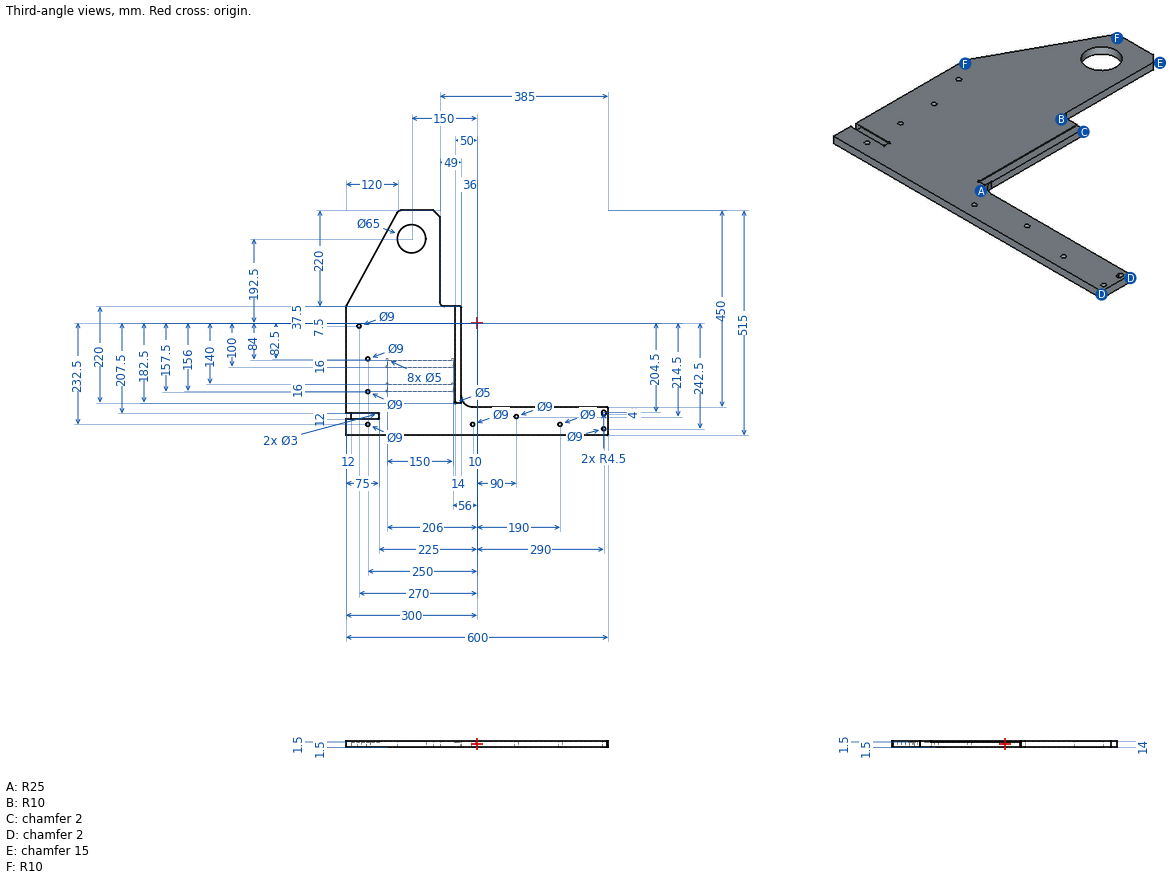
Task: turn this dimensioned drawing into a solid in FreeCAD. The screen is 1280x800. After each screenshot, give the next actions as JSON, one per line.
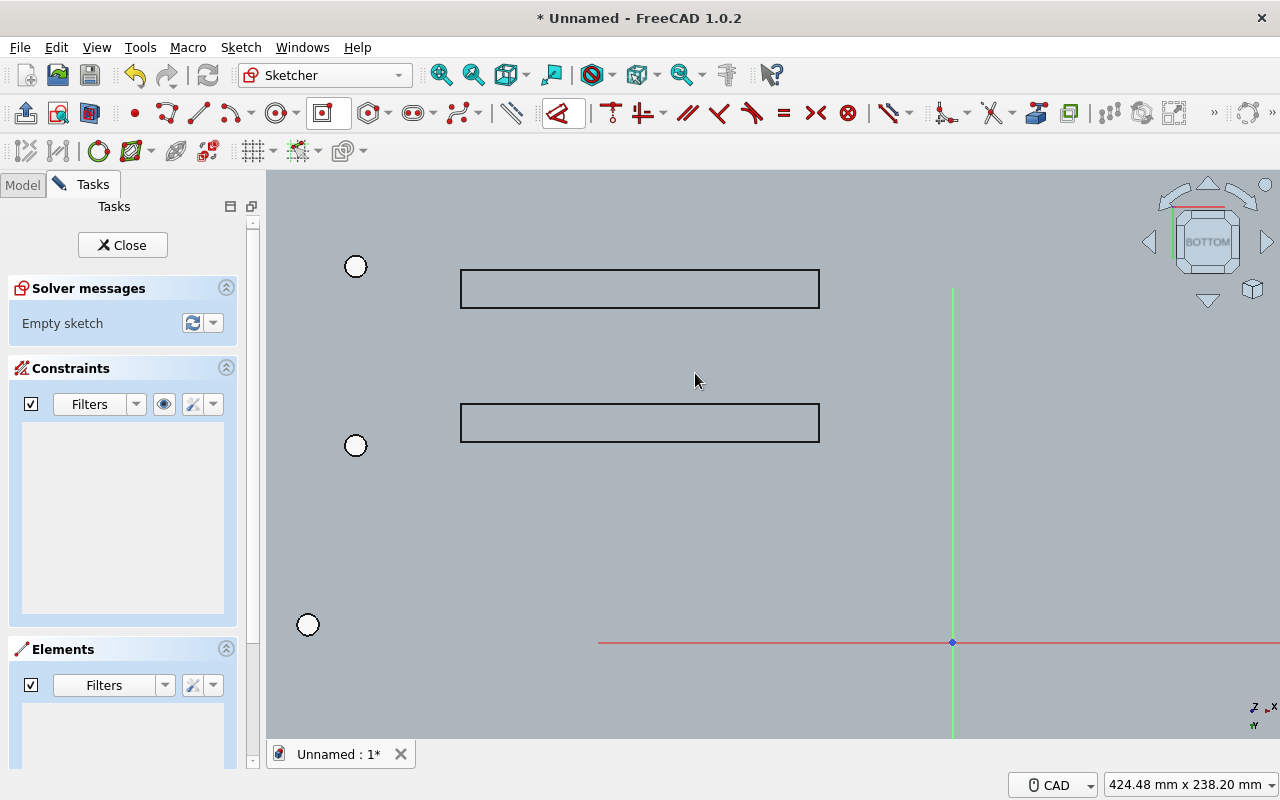
{"action": "left_click", "coordinate": [276, 114]}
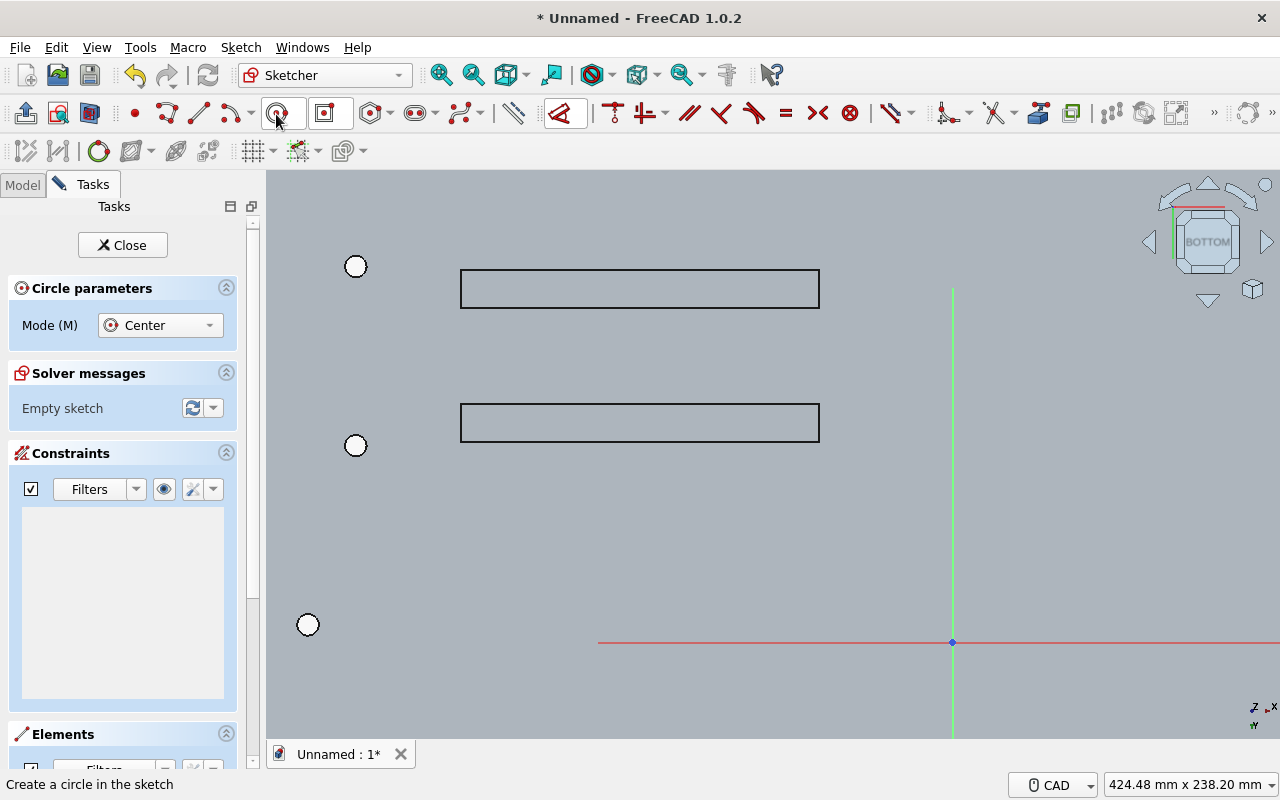
{"action": "scroll", "coordinate": [461, 442], "scroll_direction": "up", "scroll_amount": 7}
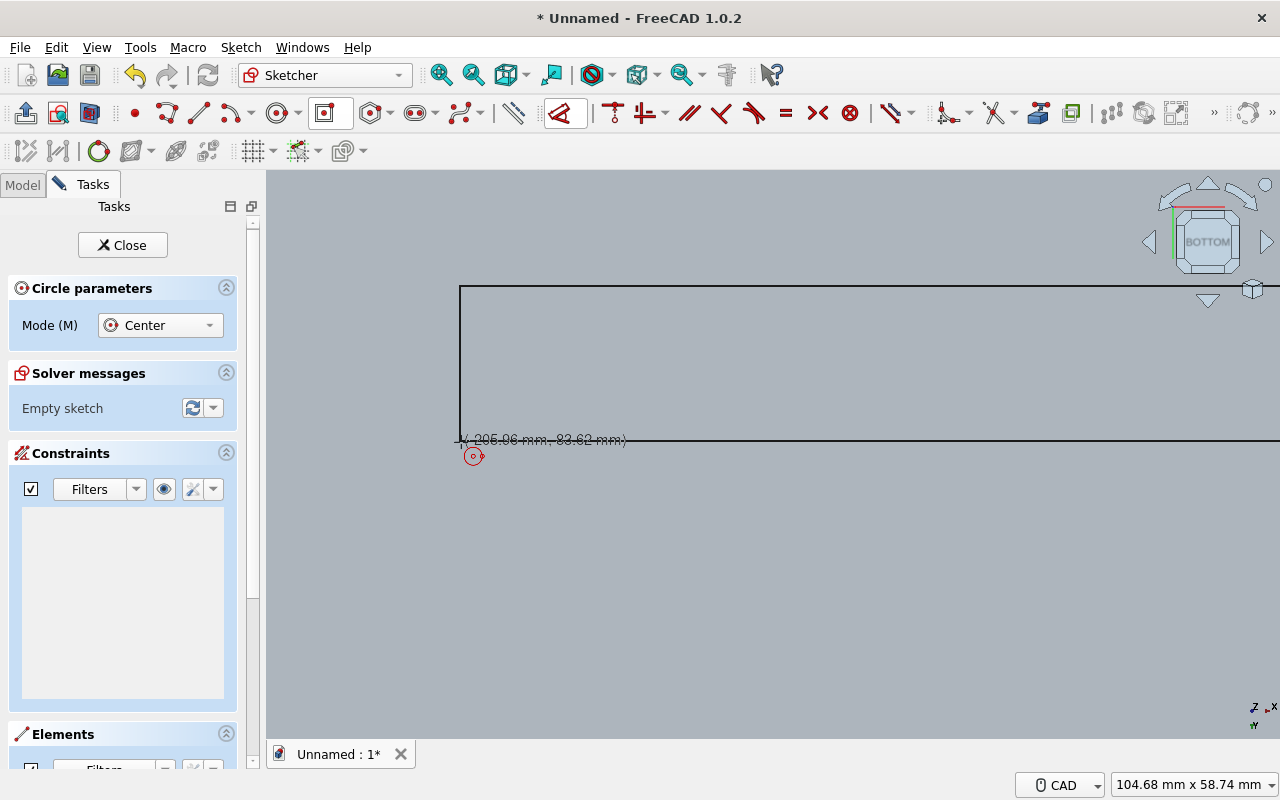
{"action": "scroll", "coordinate": [462, 444], "scroll_direction": "down", "scroll_amount": 7}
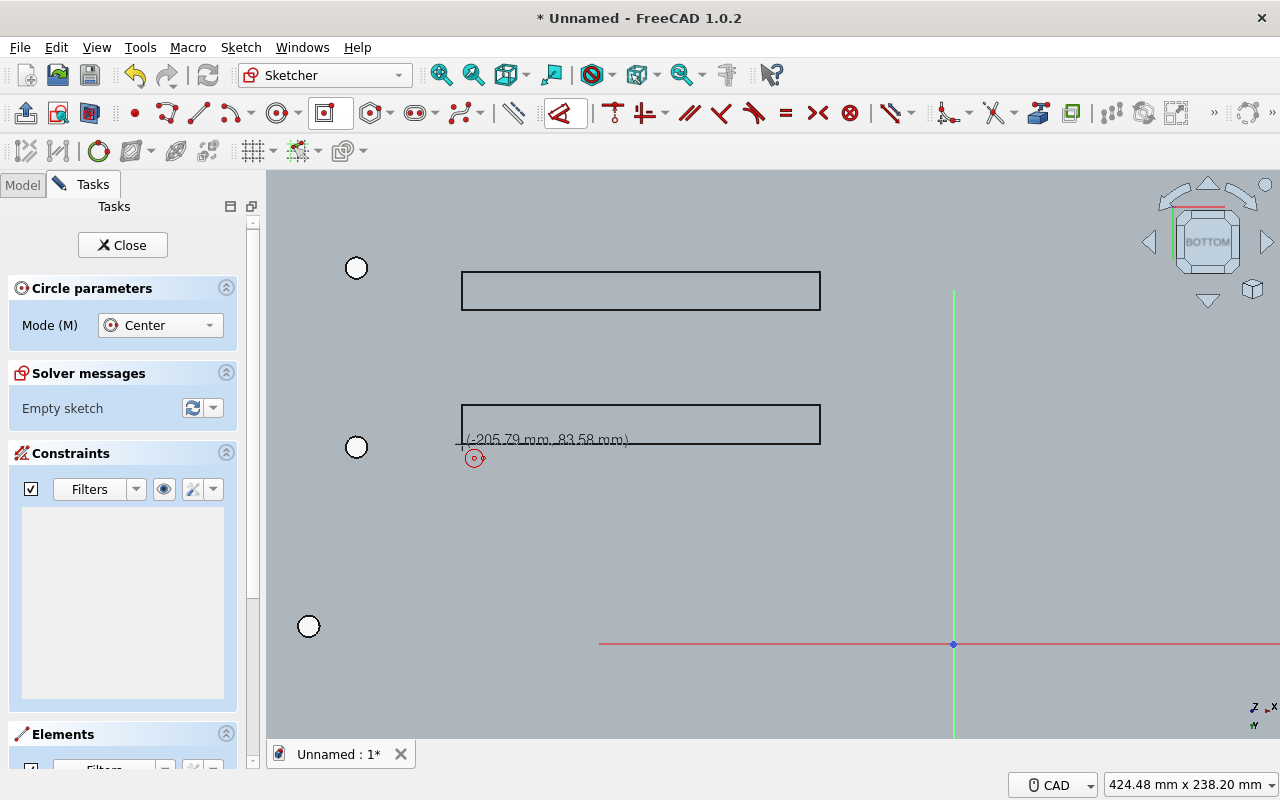
{"action": "left_click", "coordinate": [462, 444]}
{"action": "mouse_move", "coordinate": [466, 439]}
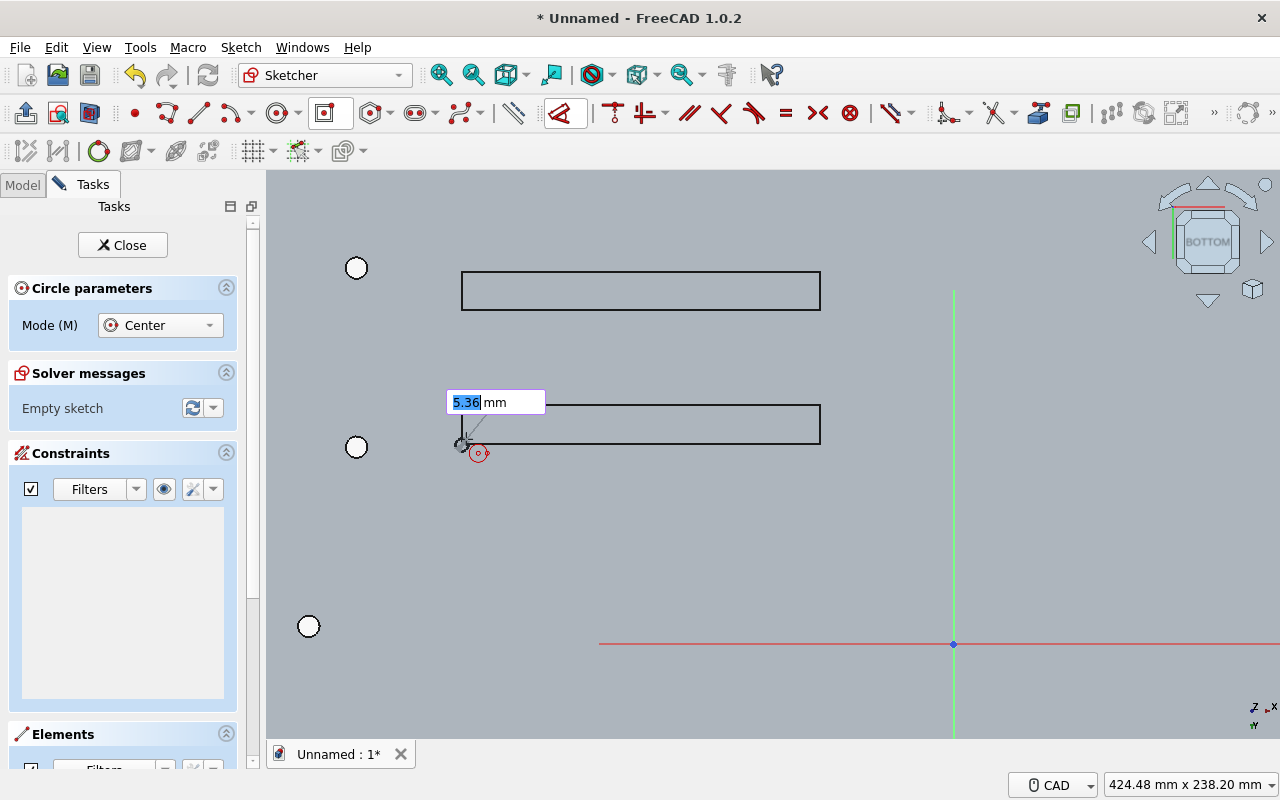
{"action": "type", "text": "5"}
{"action": "key", "text": "Return"}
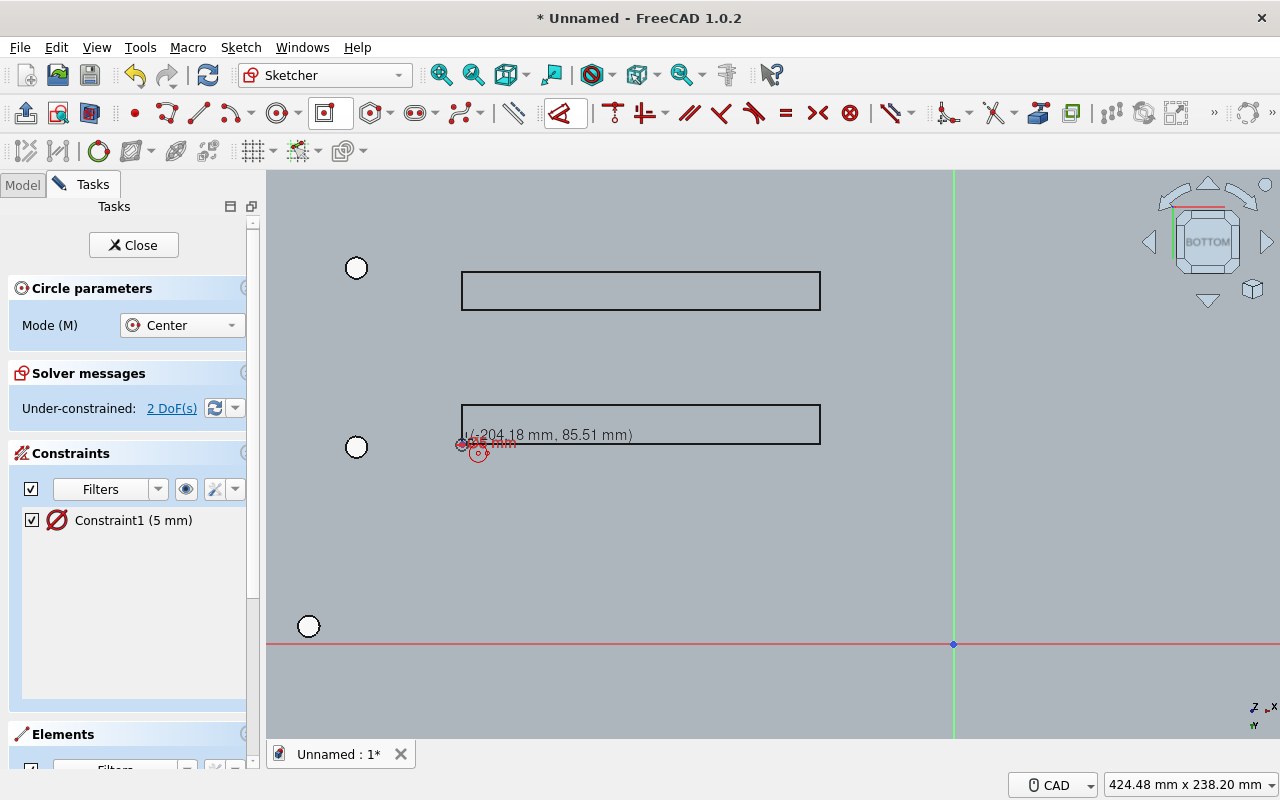
{"action": "scroll", "coordinate": [462, 405], "scroll_direction": "up", "scroll_amount": 7}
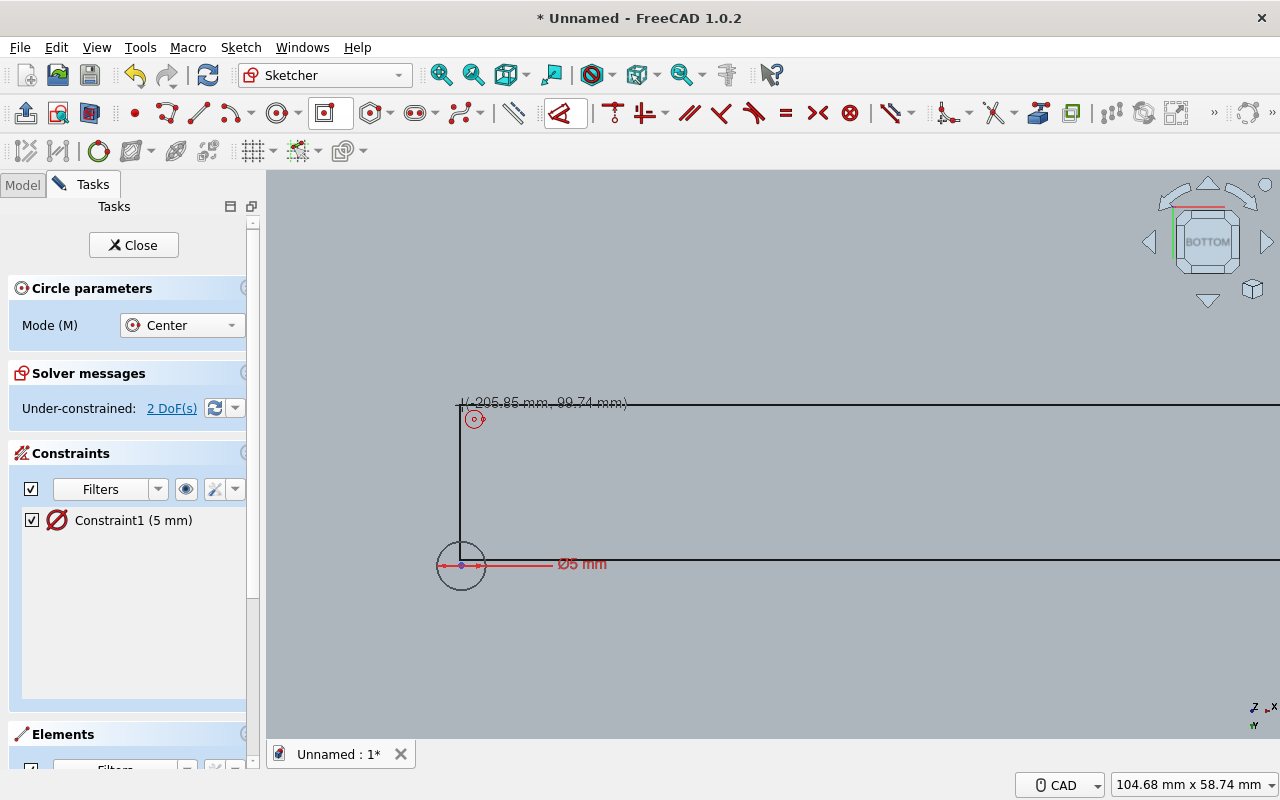
{"action": "scroll", "coordinate": [462, 405], "scroll_direction": "down", "scroll_amount": 7}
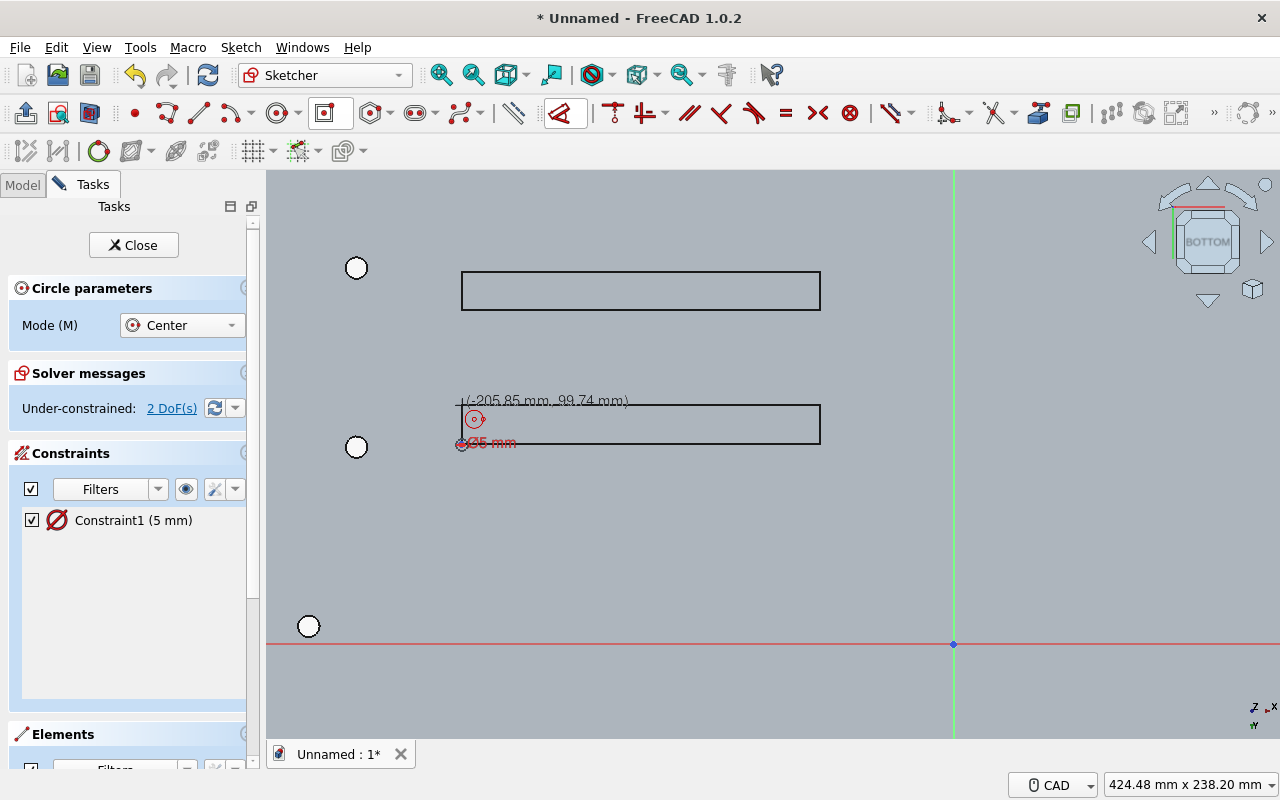
{"action": "left_click", "coordinate": [462, 405]}
{"action": "mouse_move", "coordinate": [466, 401]}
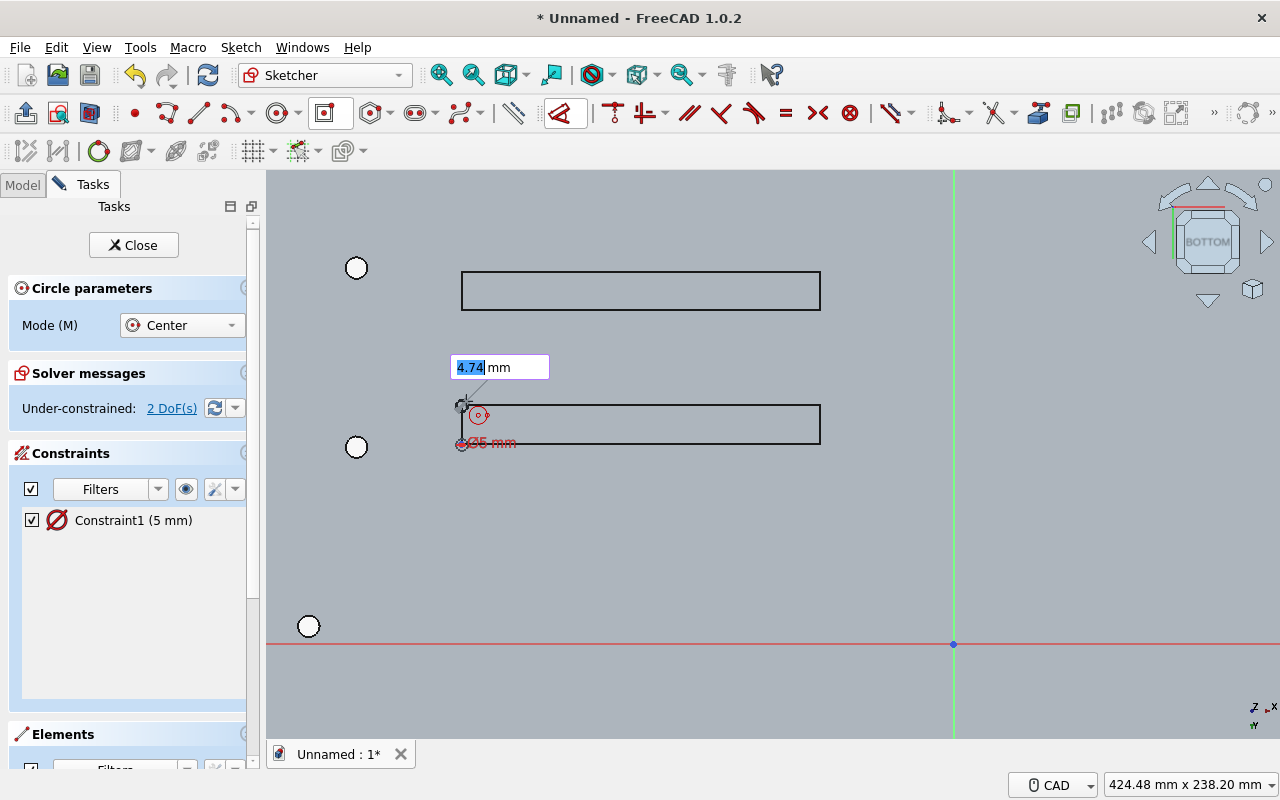
{"action": "type", "text": "5"}
{"action": "key", "text": "Return"}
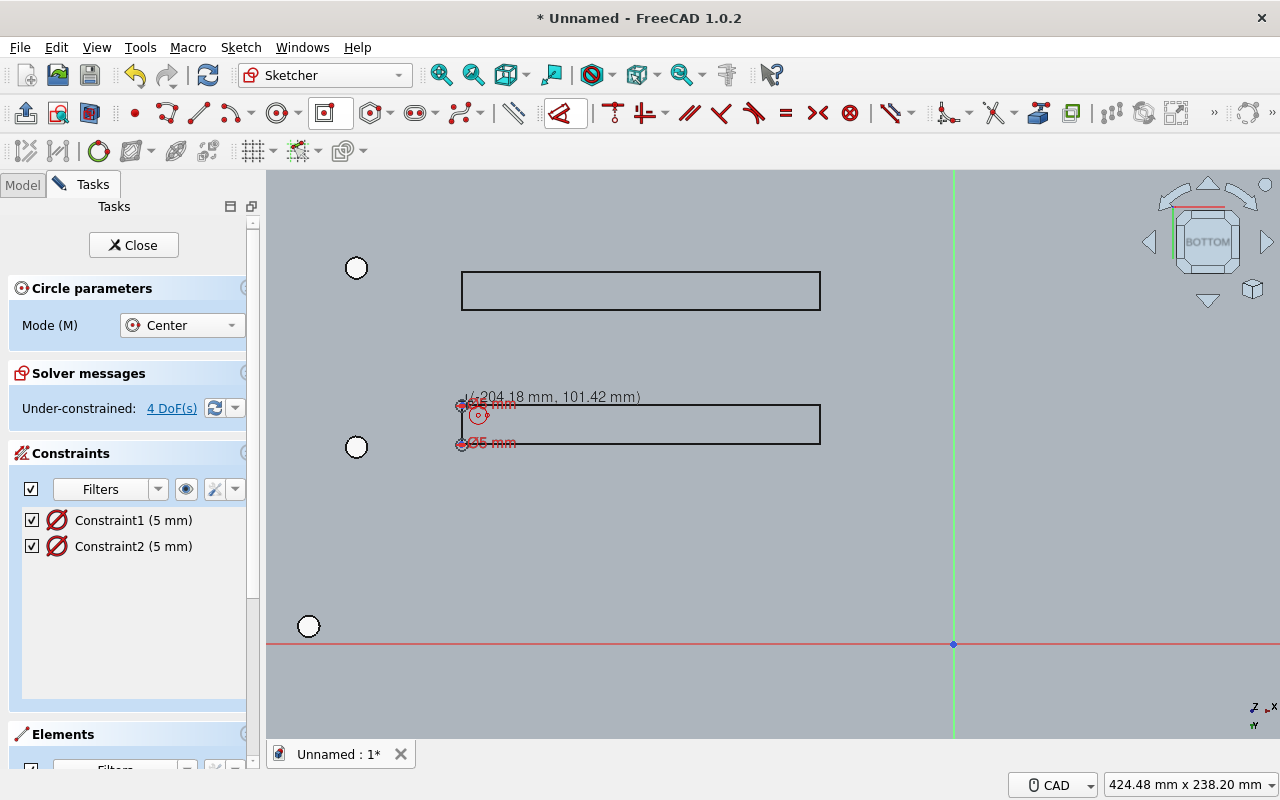
{"action": "scroll", "coordinate": [462, 310], "scroll_direction": "up", "scroll_amount": 7}